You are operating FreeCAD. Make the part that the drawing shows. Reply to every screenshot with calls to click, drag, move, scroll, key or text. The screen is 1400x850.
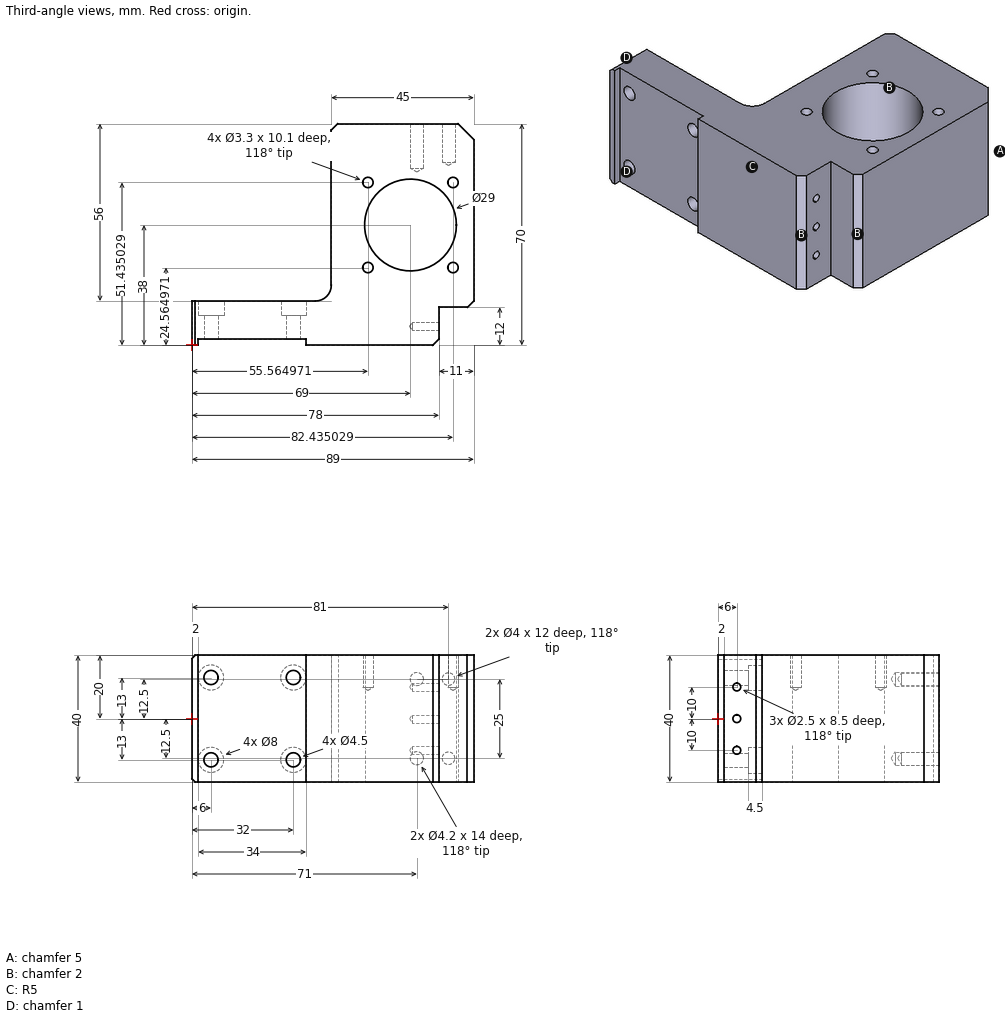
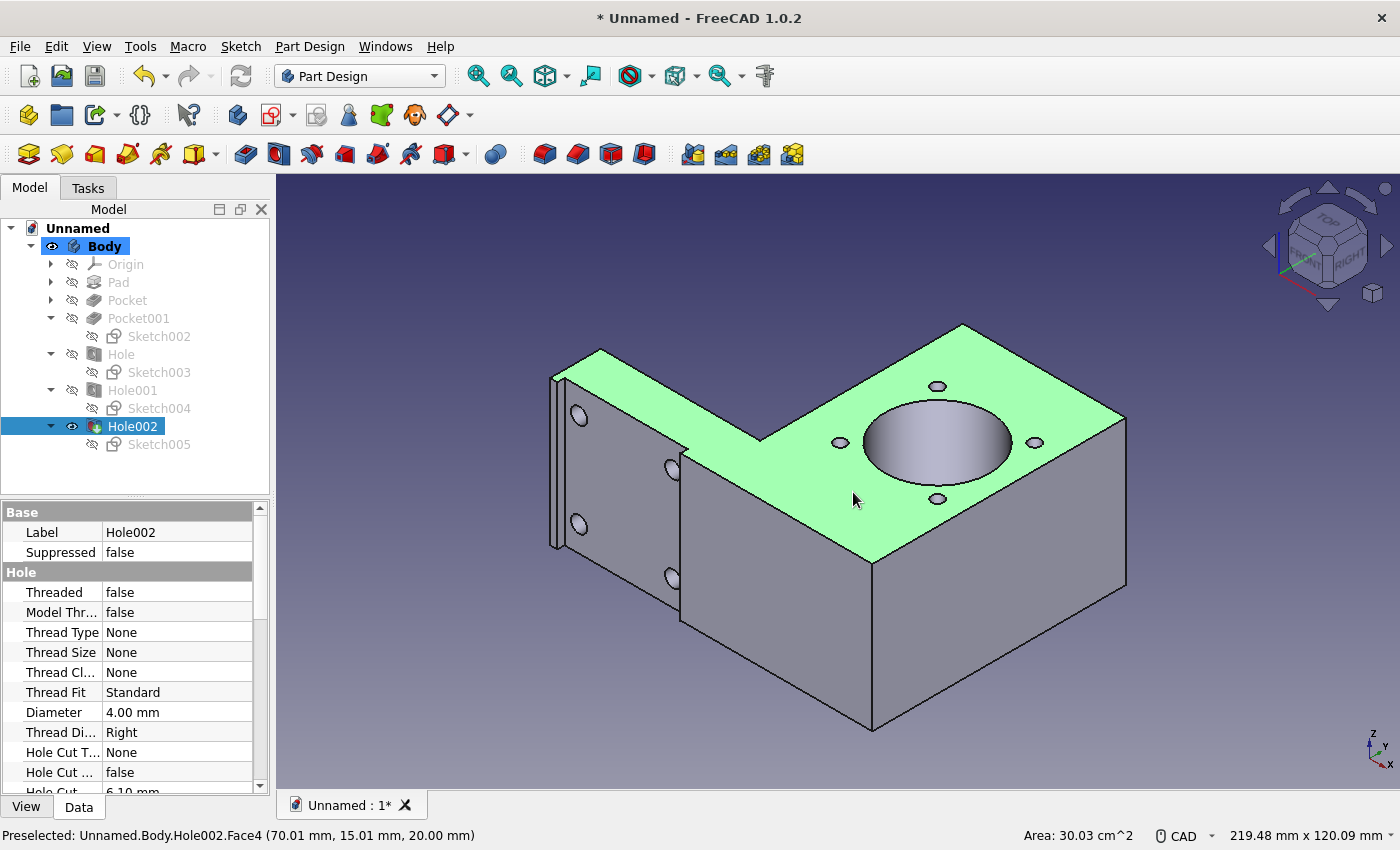
click(270, 116)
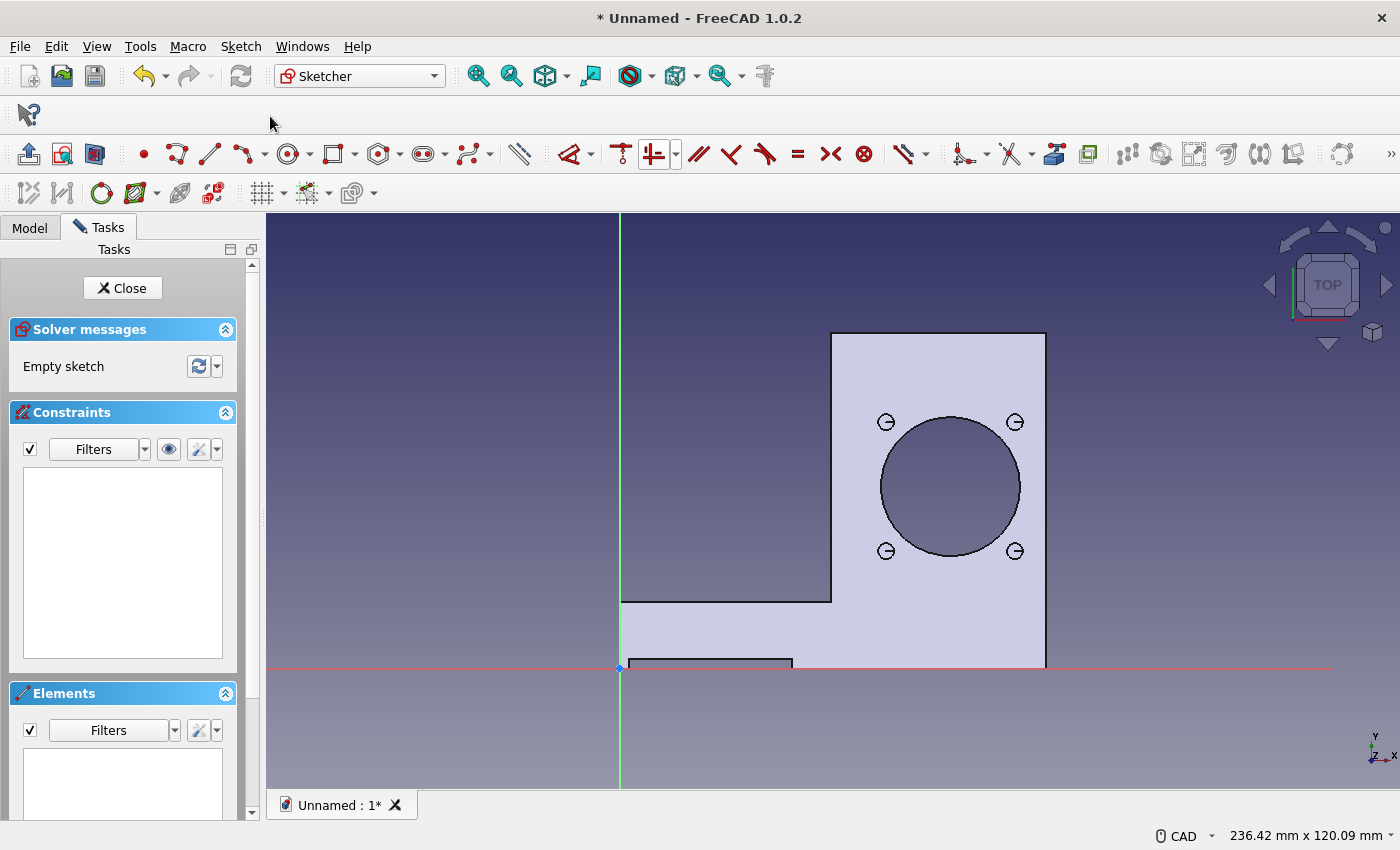
scroll(1071, 668, up, 9)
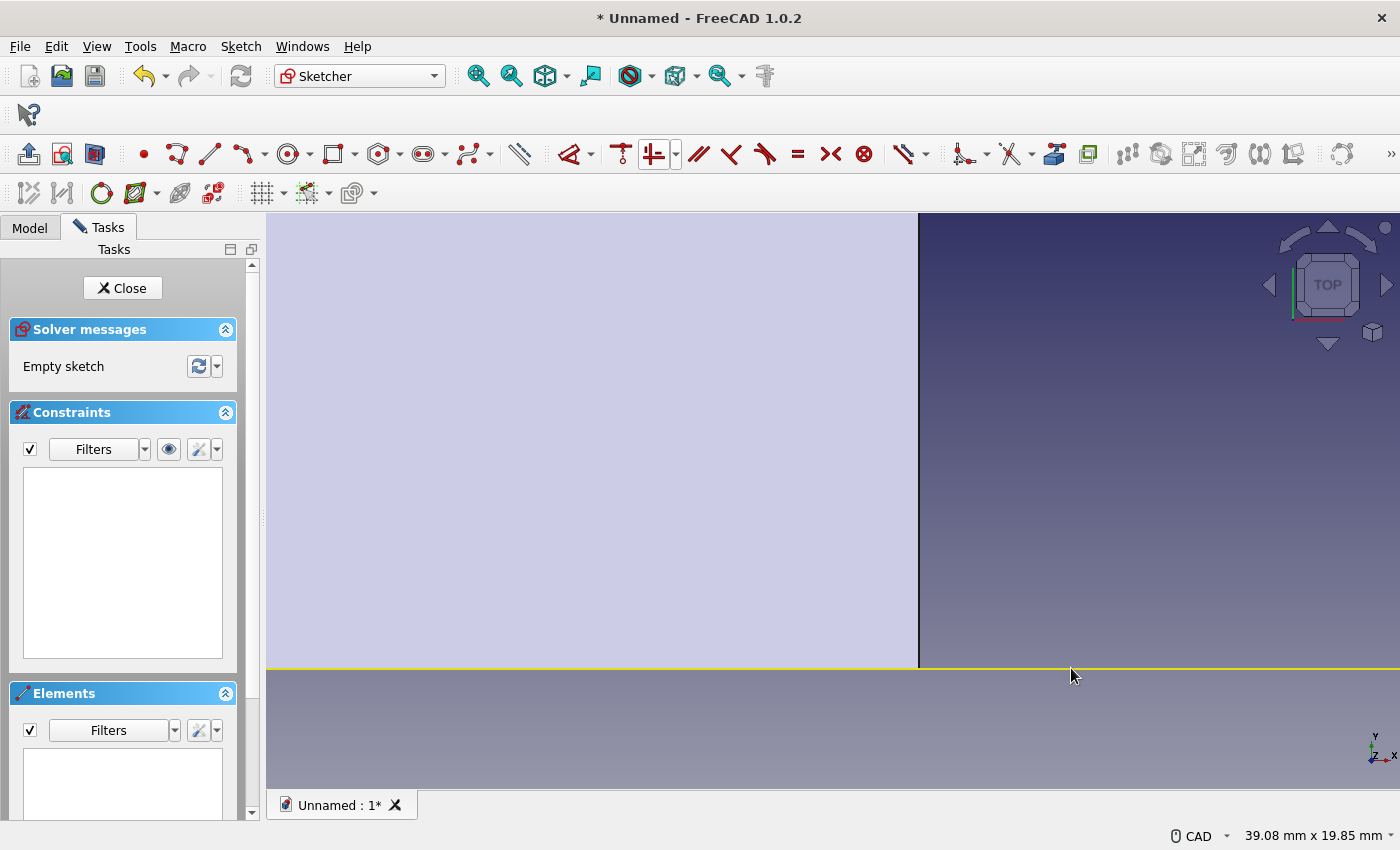
click(332, 154)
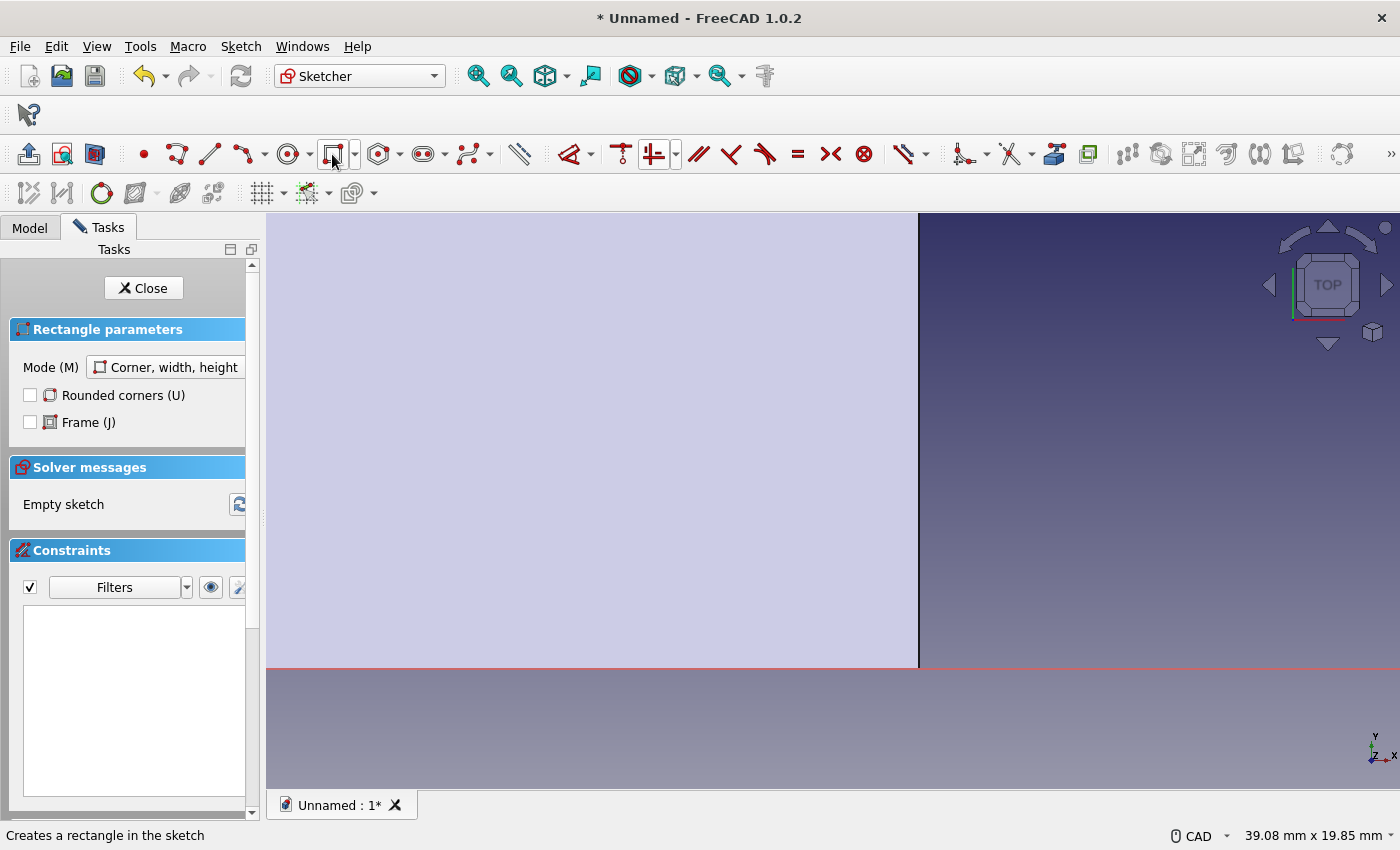
click(600, 321)
click(919, 669)
key(Escape)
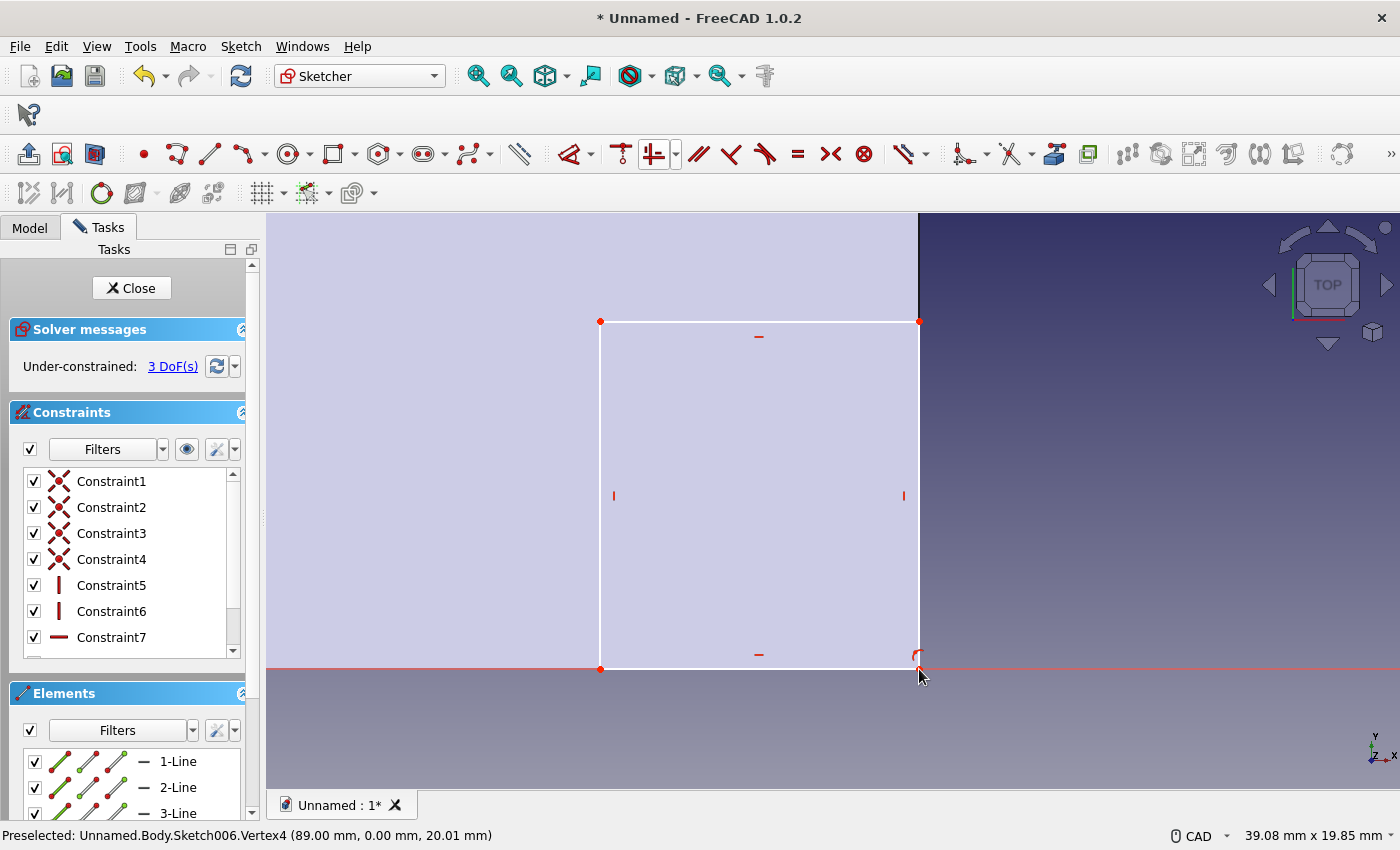
key(d)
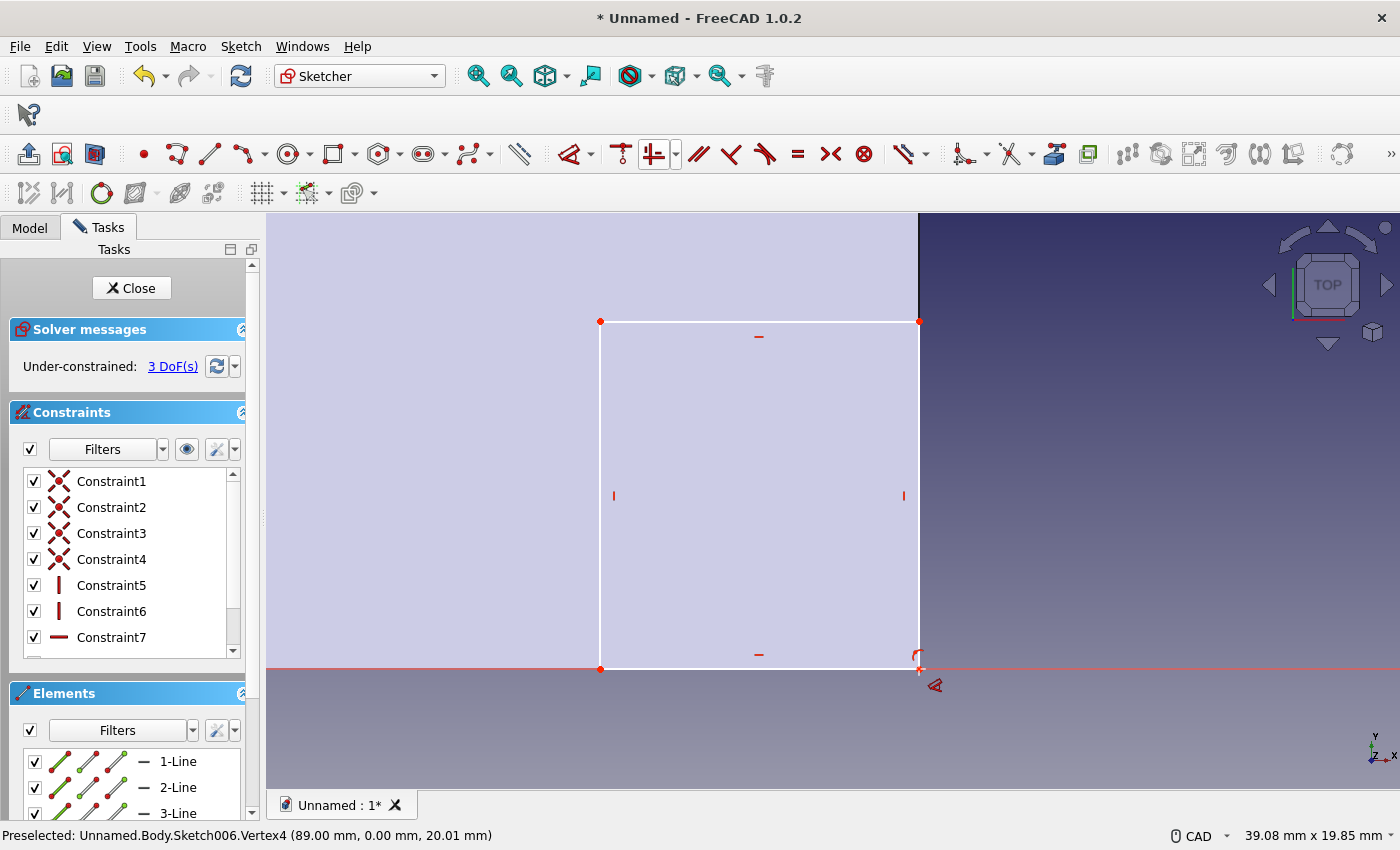
click(600, 426)
click(566, 496)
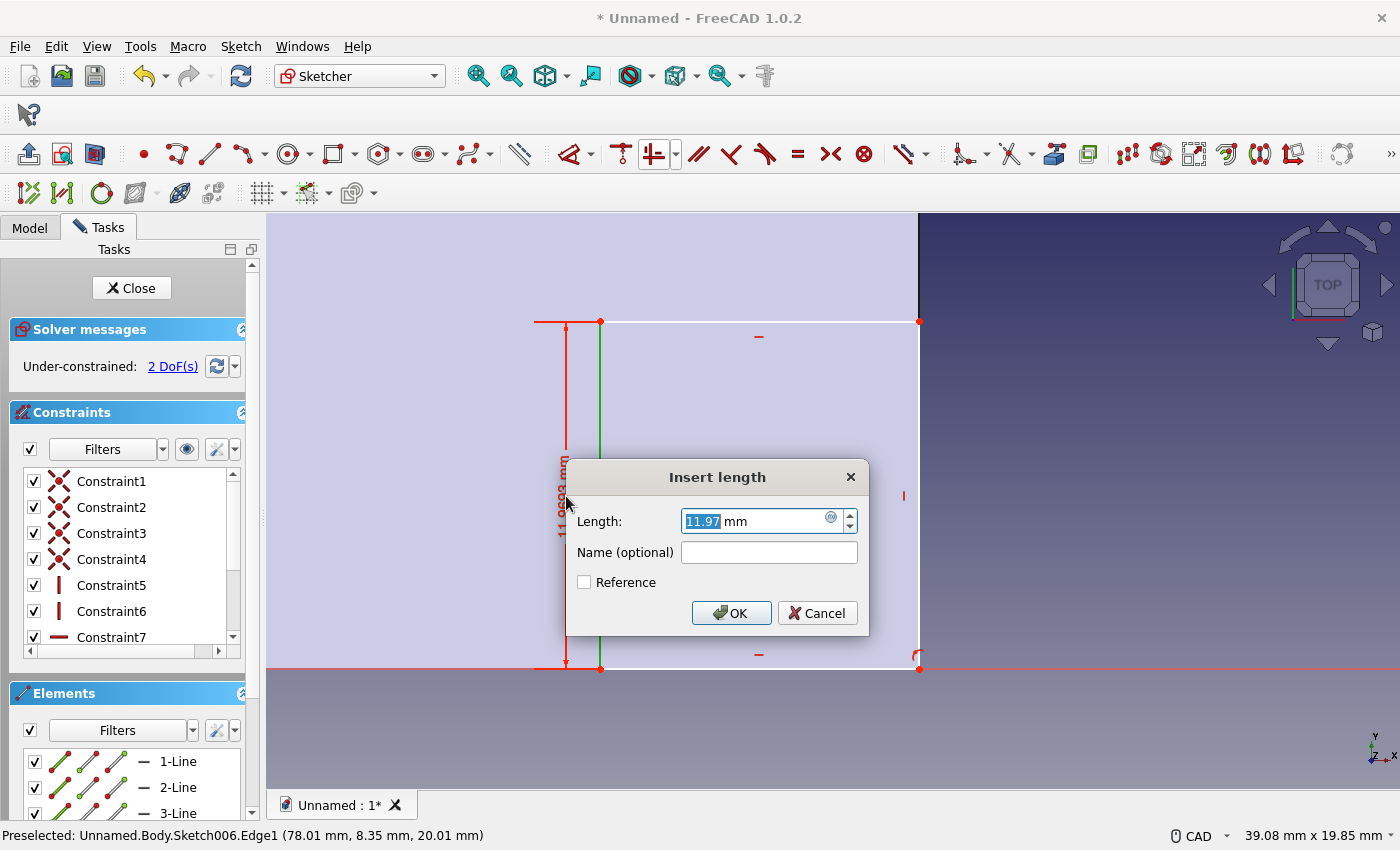
text(12)
key(Return)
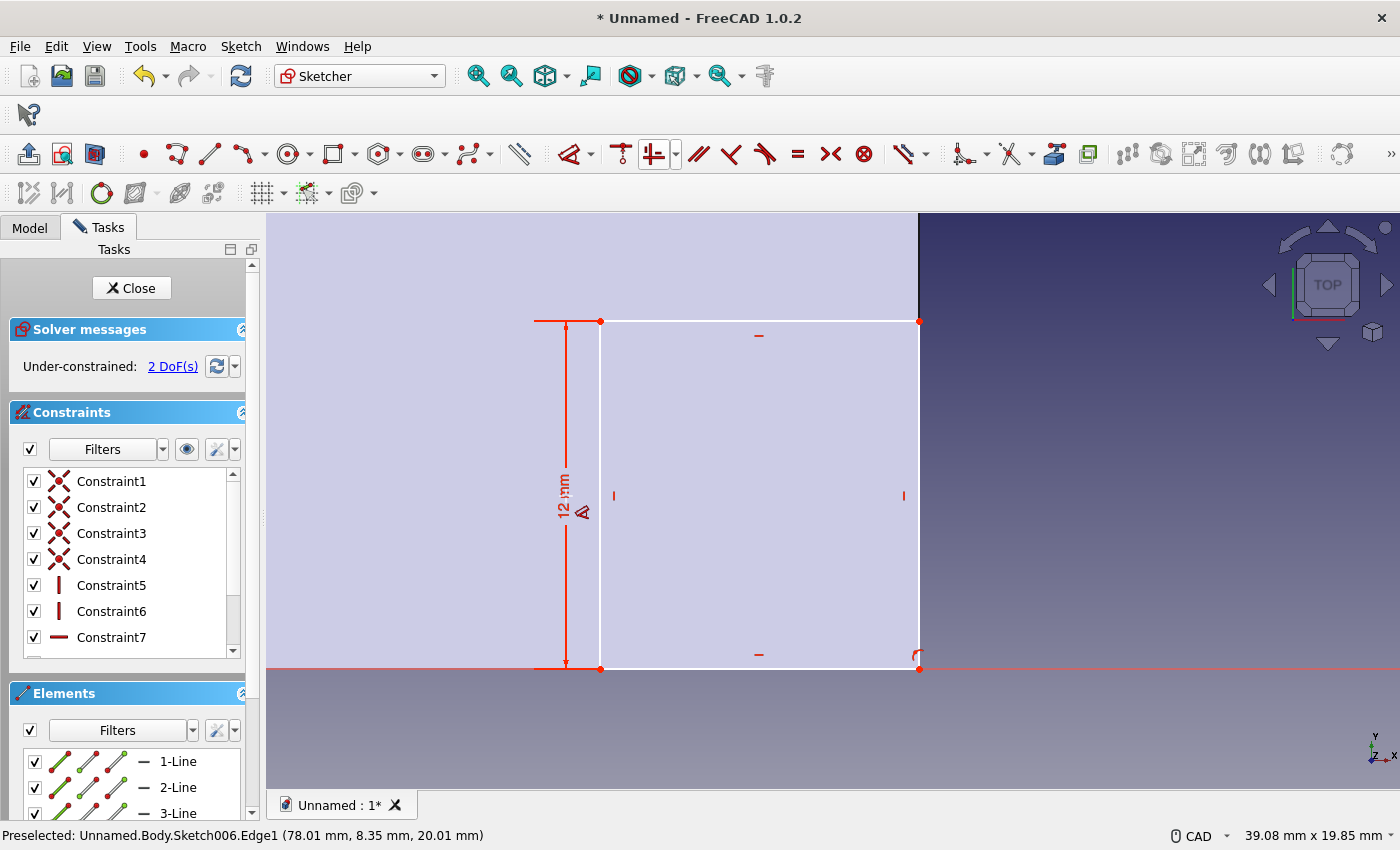
click(696, 669)
click(759, 703)